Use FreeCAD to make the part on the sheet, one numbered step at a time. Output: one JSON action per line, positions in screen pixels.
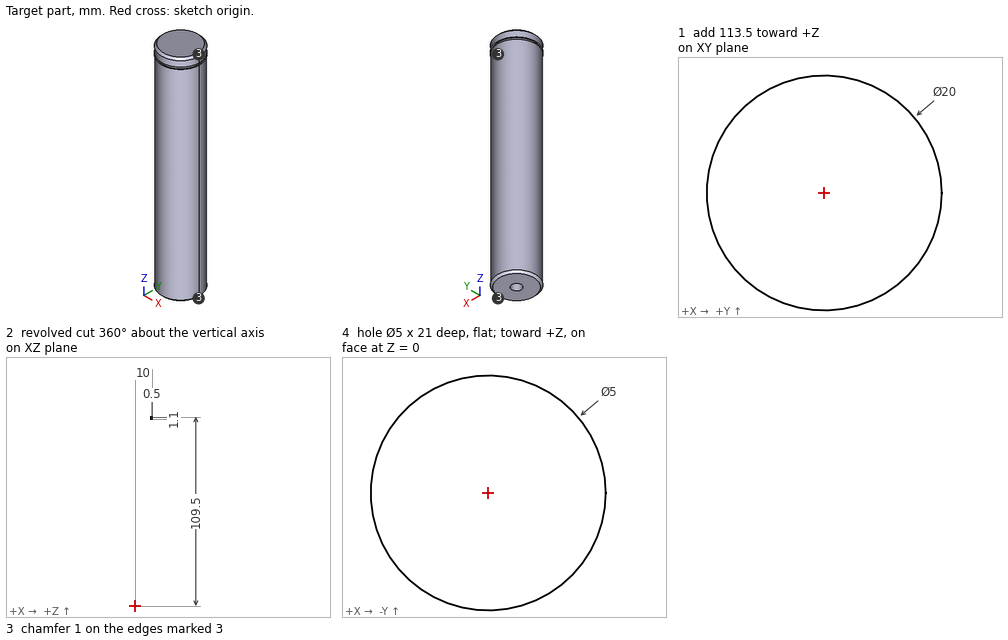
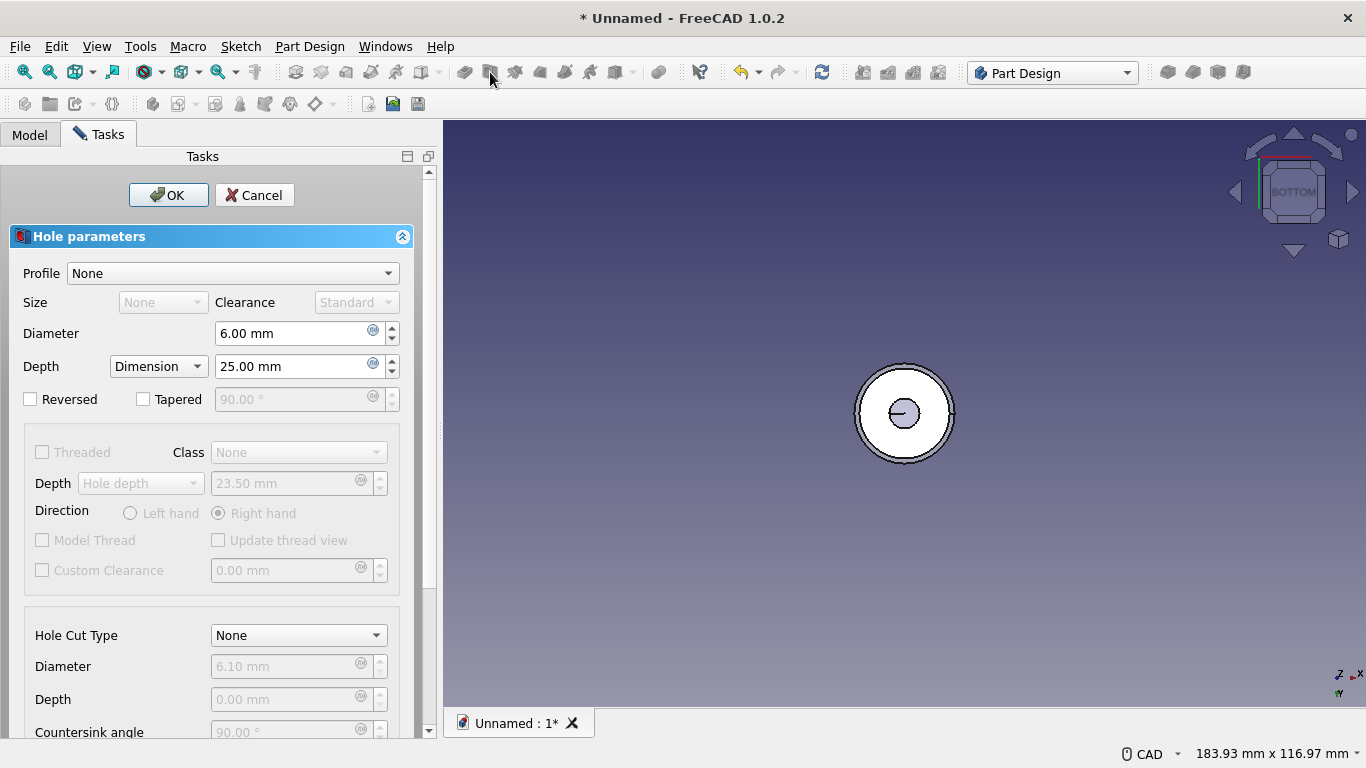
{"action": "triple_click", "coordinate": [300, 334]}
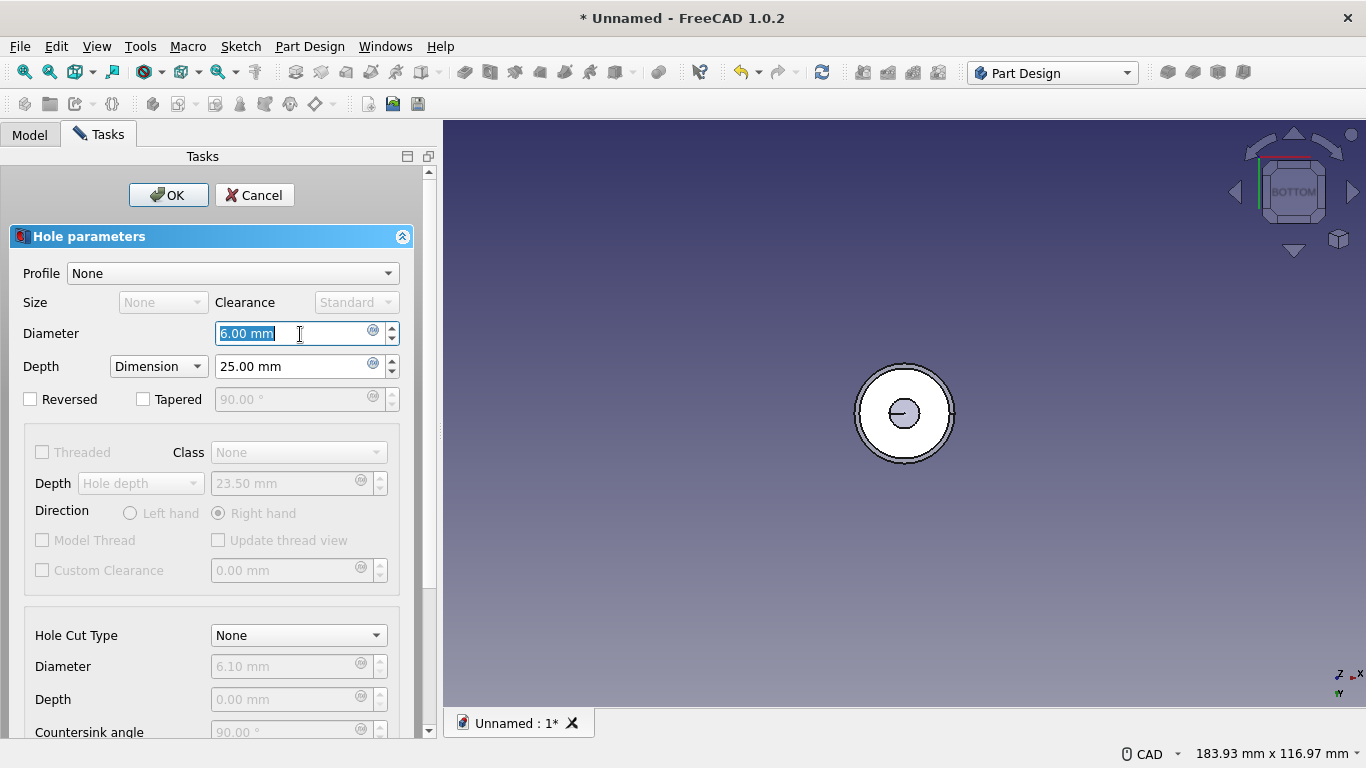
{"action": "type", "text": "5"}
{"action": "key", "text": "Tab"}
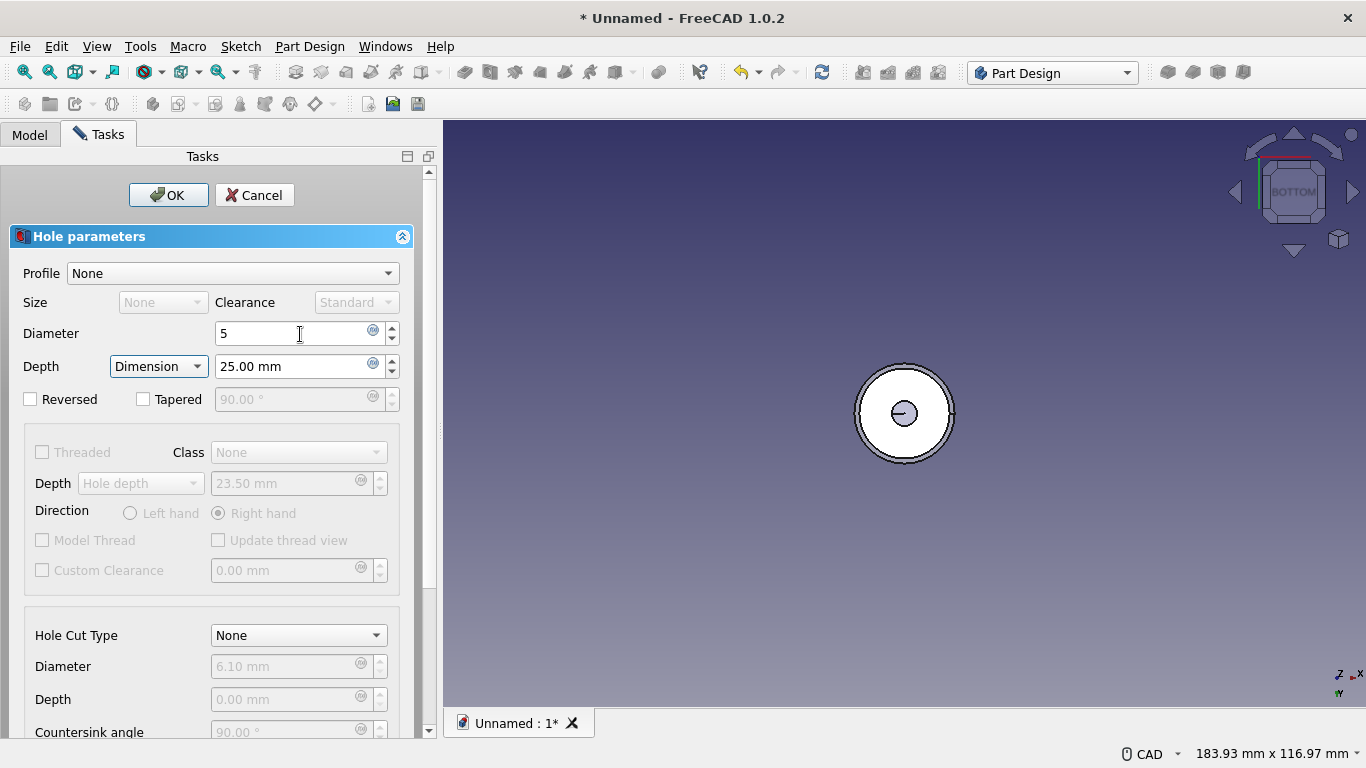
{"action": "triple_click", "coordinate": [300, 366]}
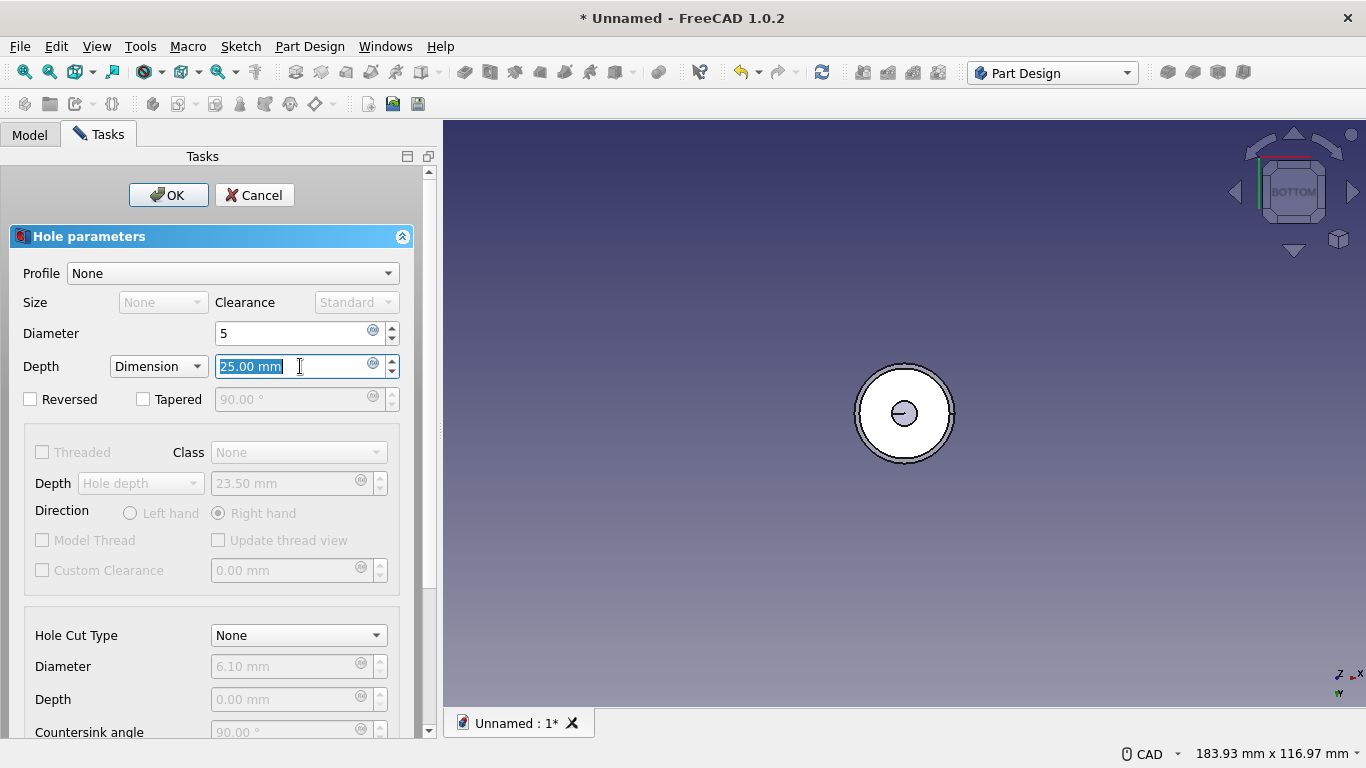
{"action": "type", "text": "21"}
{"action": "key", "text": "Tab"}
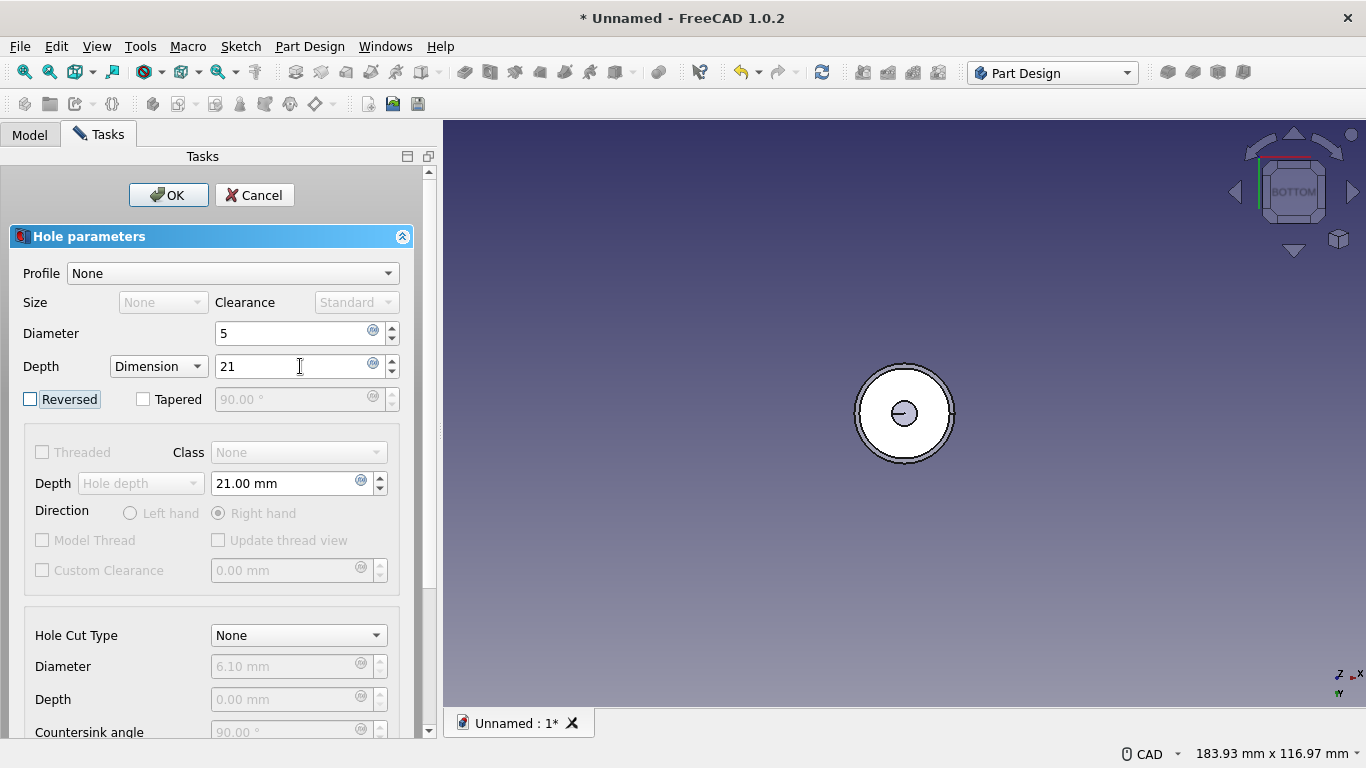
{"action": "scroll", "coordinate": [429, 452], "scroll_direction": "down", "scroll_amount": 3}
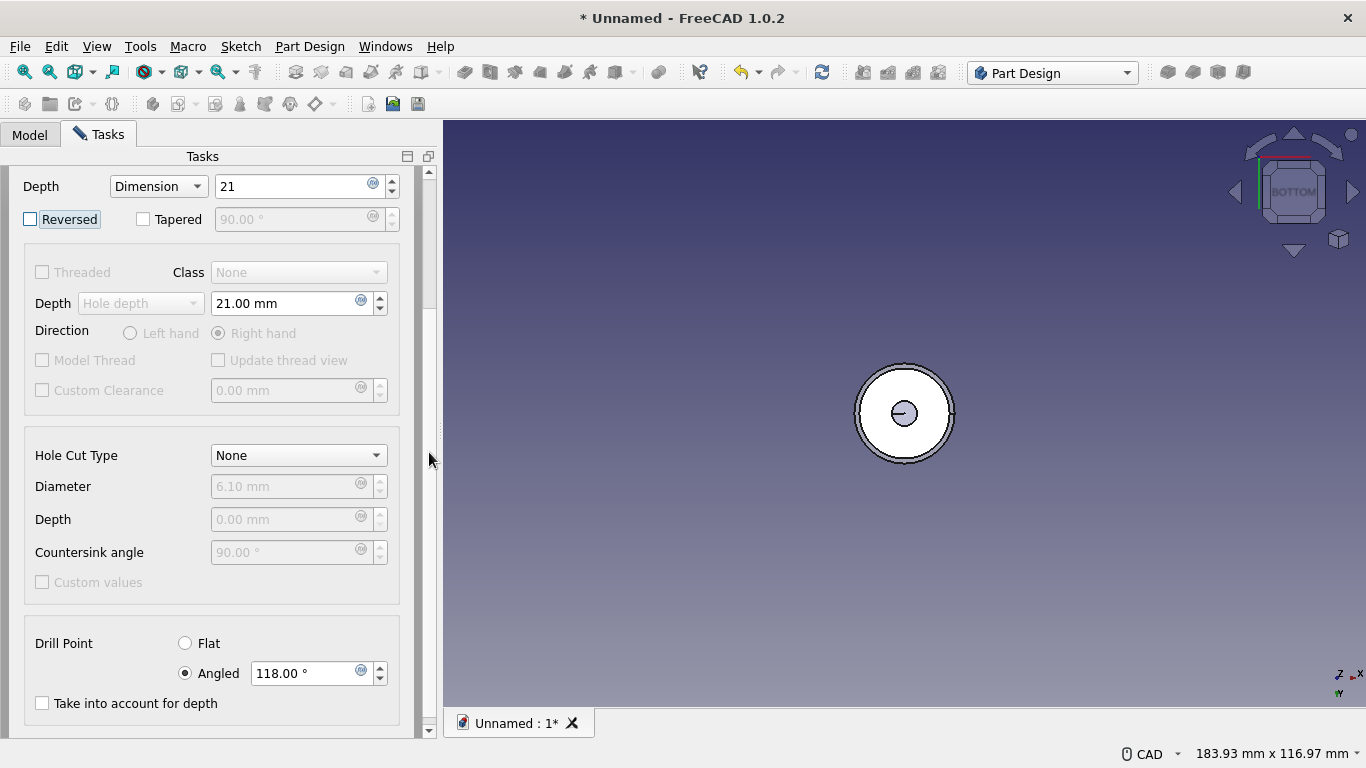
{"action": "left_click", "coordinate": [186, 641]}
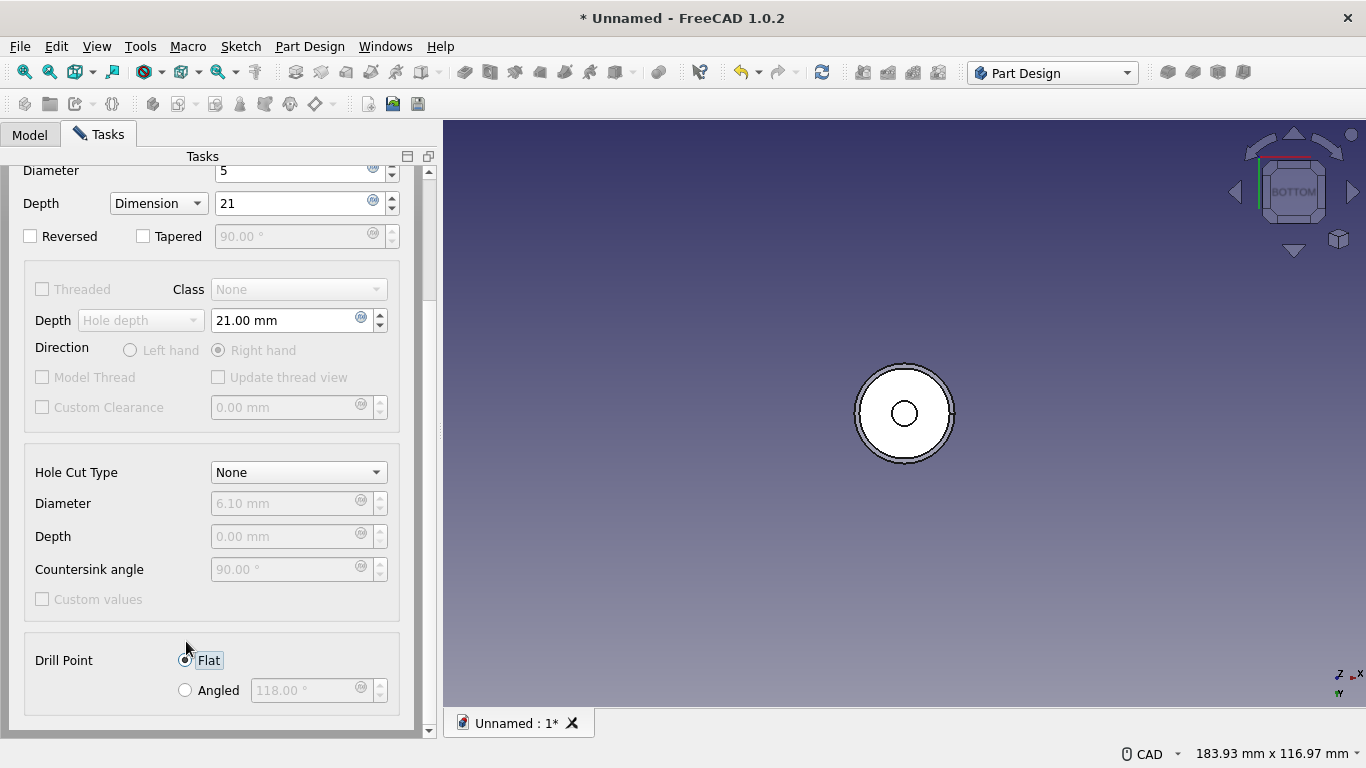
{"action": "scroll", "coordinate": [429, 452], "scroll_direction": "up", "scroll_amount": 4}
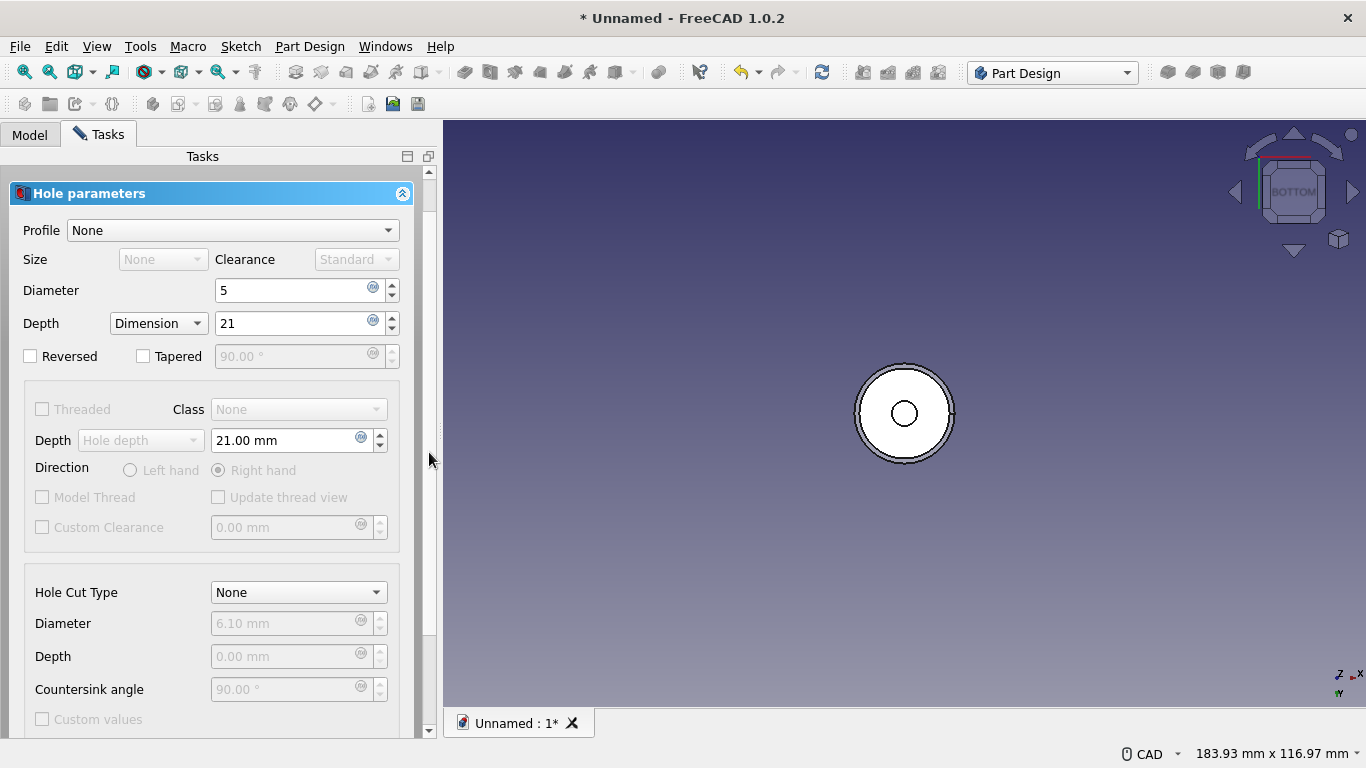
{"action": "left_click", "coordinate": [169, 195]}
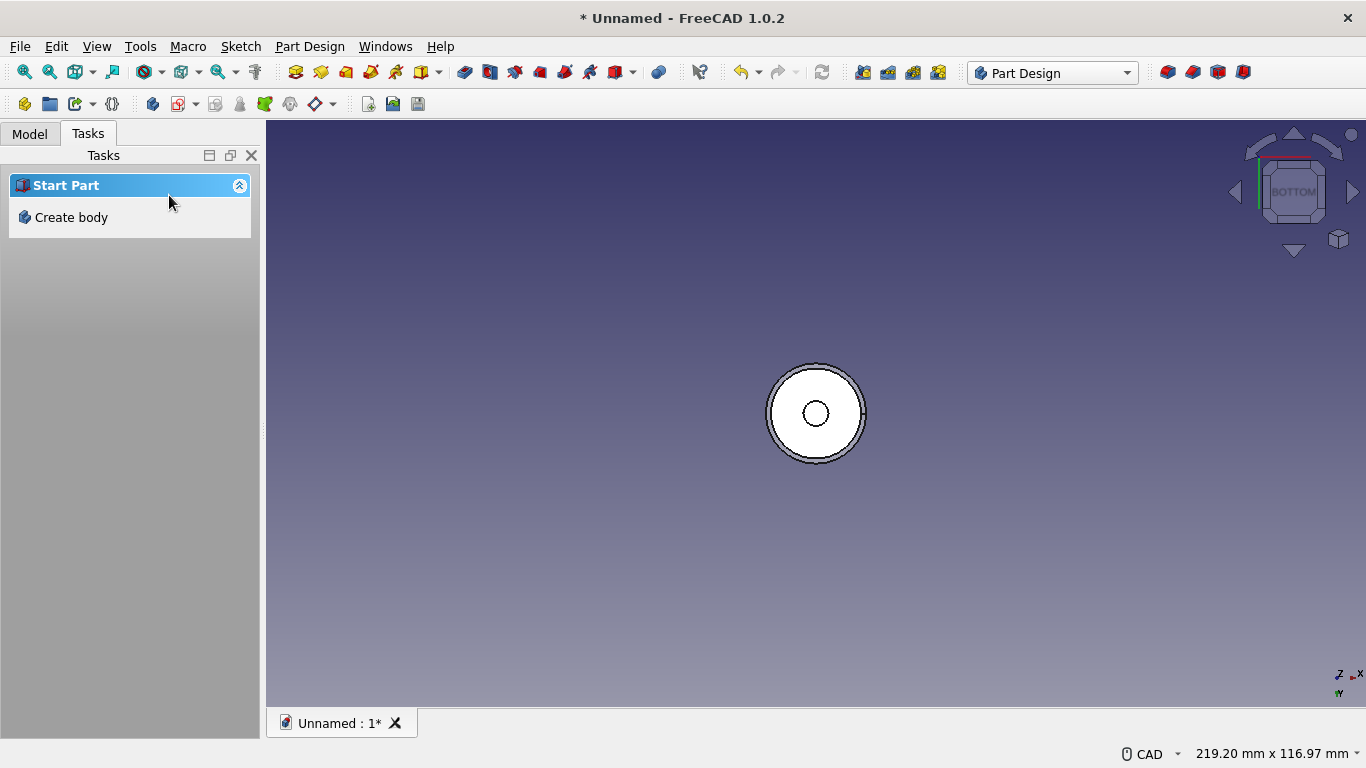
{"action": "key", "text": "0"}